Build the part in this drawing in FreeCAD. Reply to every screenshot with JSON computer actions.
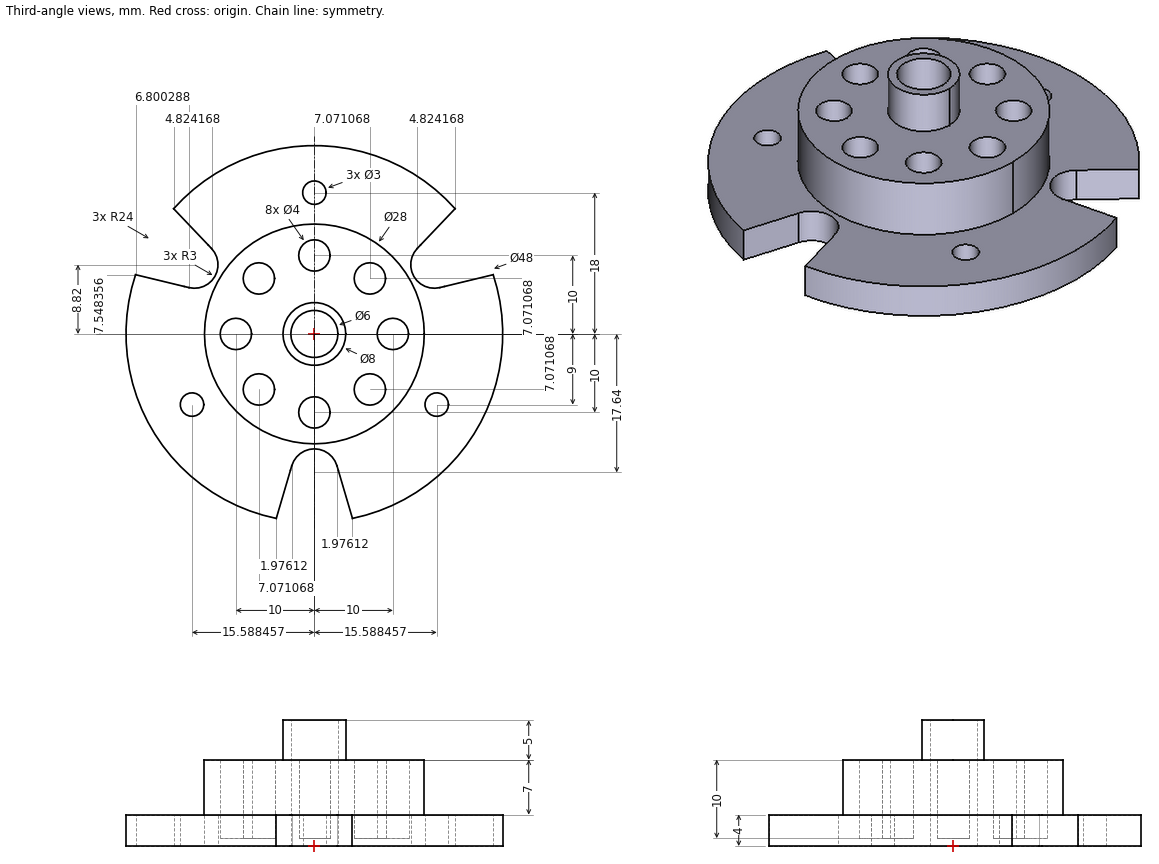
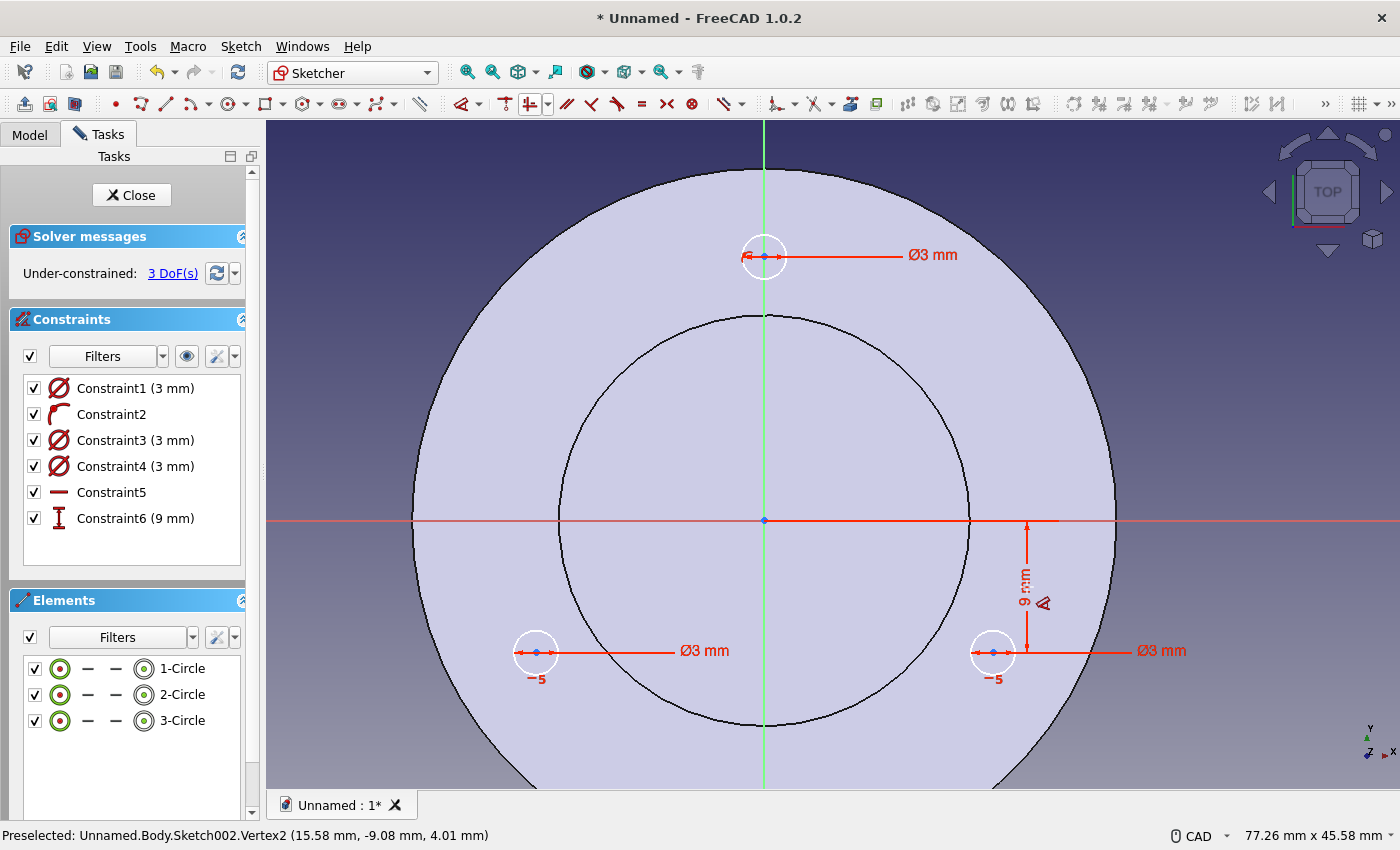
{"action": "left_click", "coordinate": [764, 257]}
{"action": "left_click", "coordinate": [798, 389]}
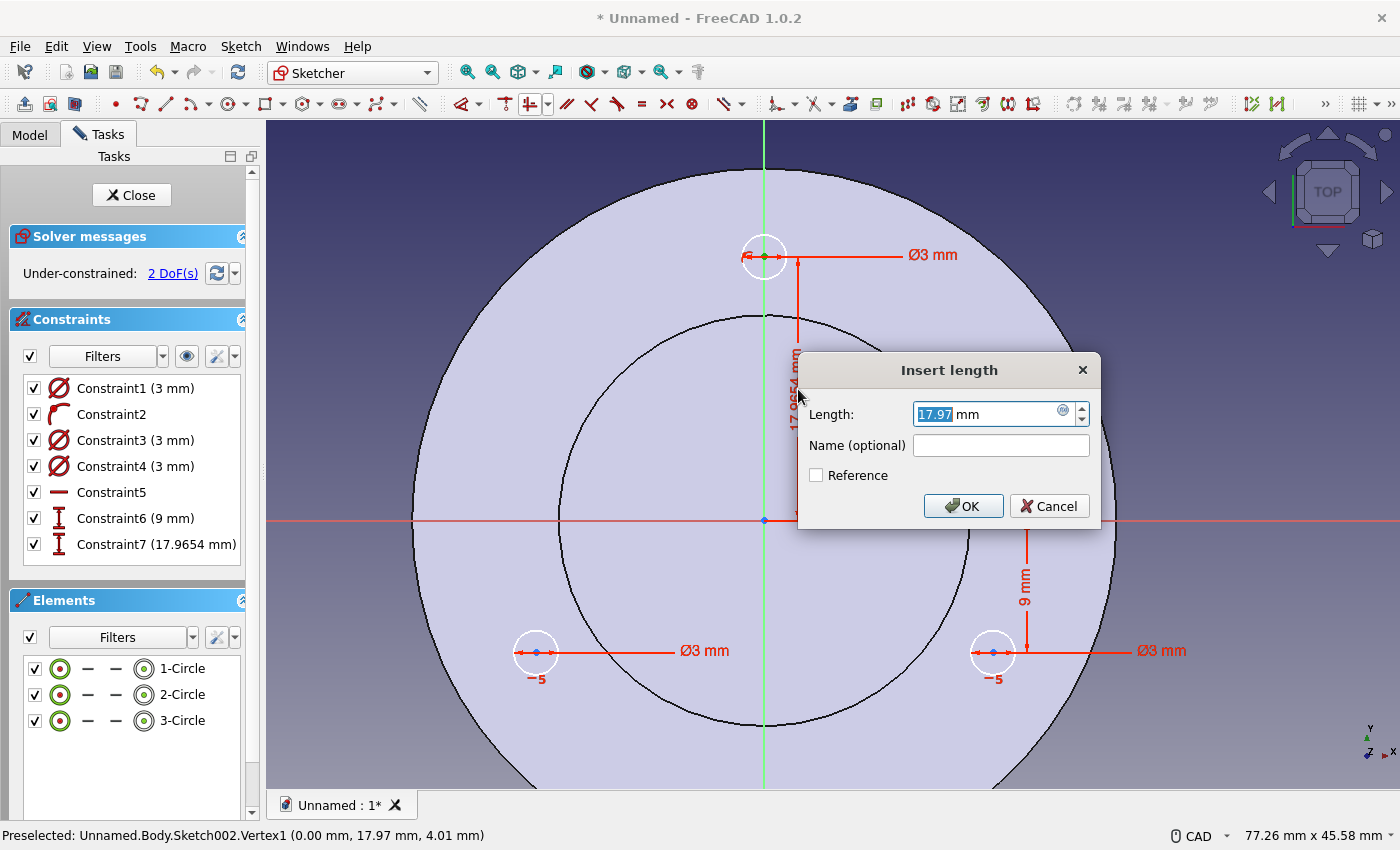
{"action": "type", "text": "18"}
{"action": "key", "text": "Return"}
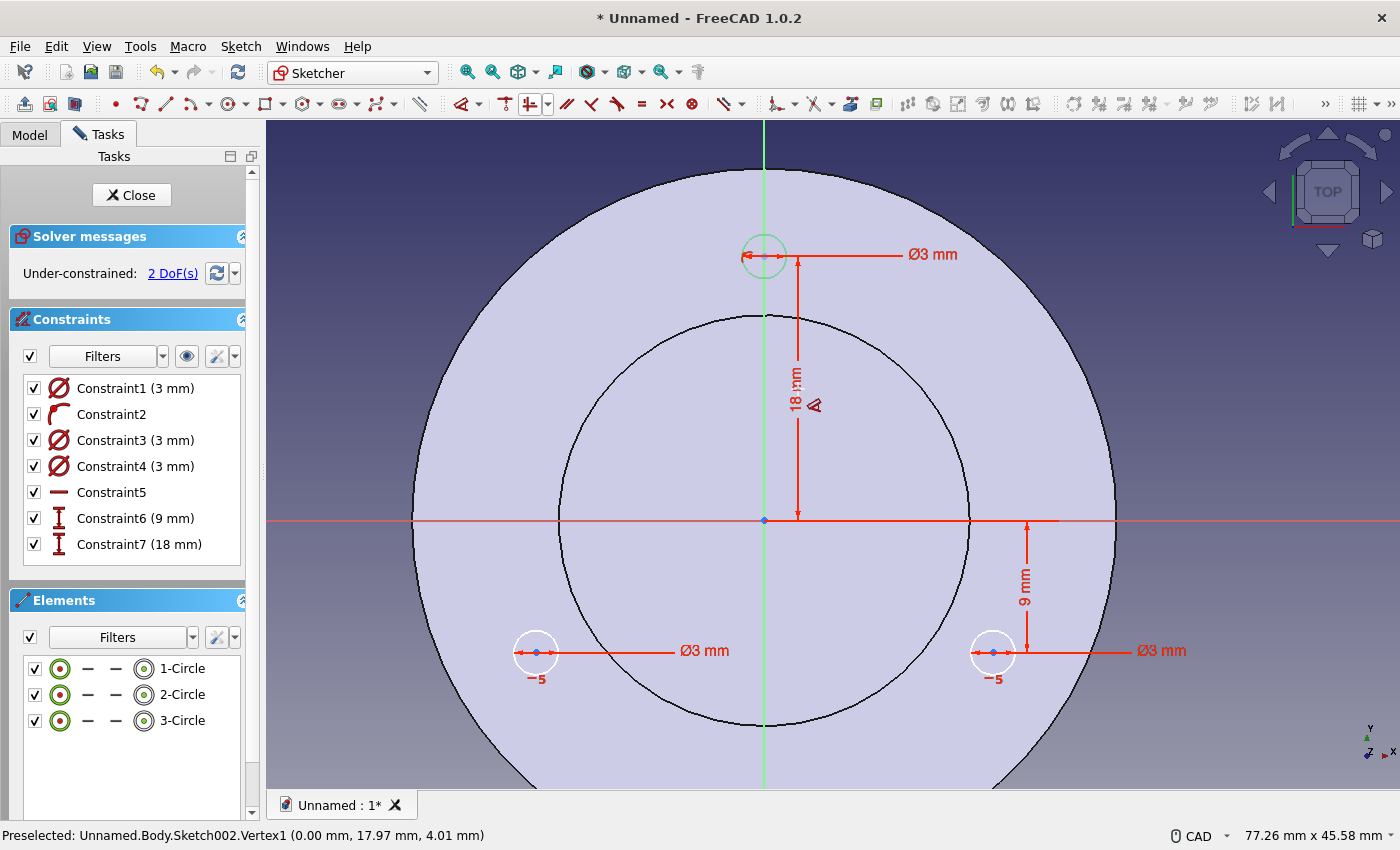
{"action": "left_click", "coordinate": [993, 653]}
{"action": "left_click", "coordinate": [879, 687]}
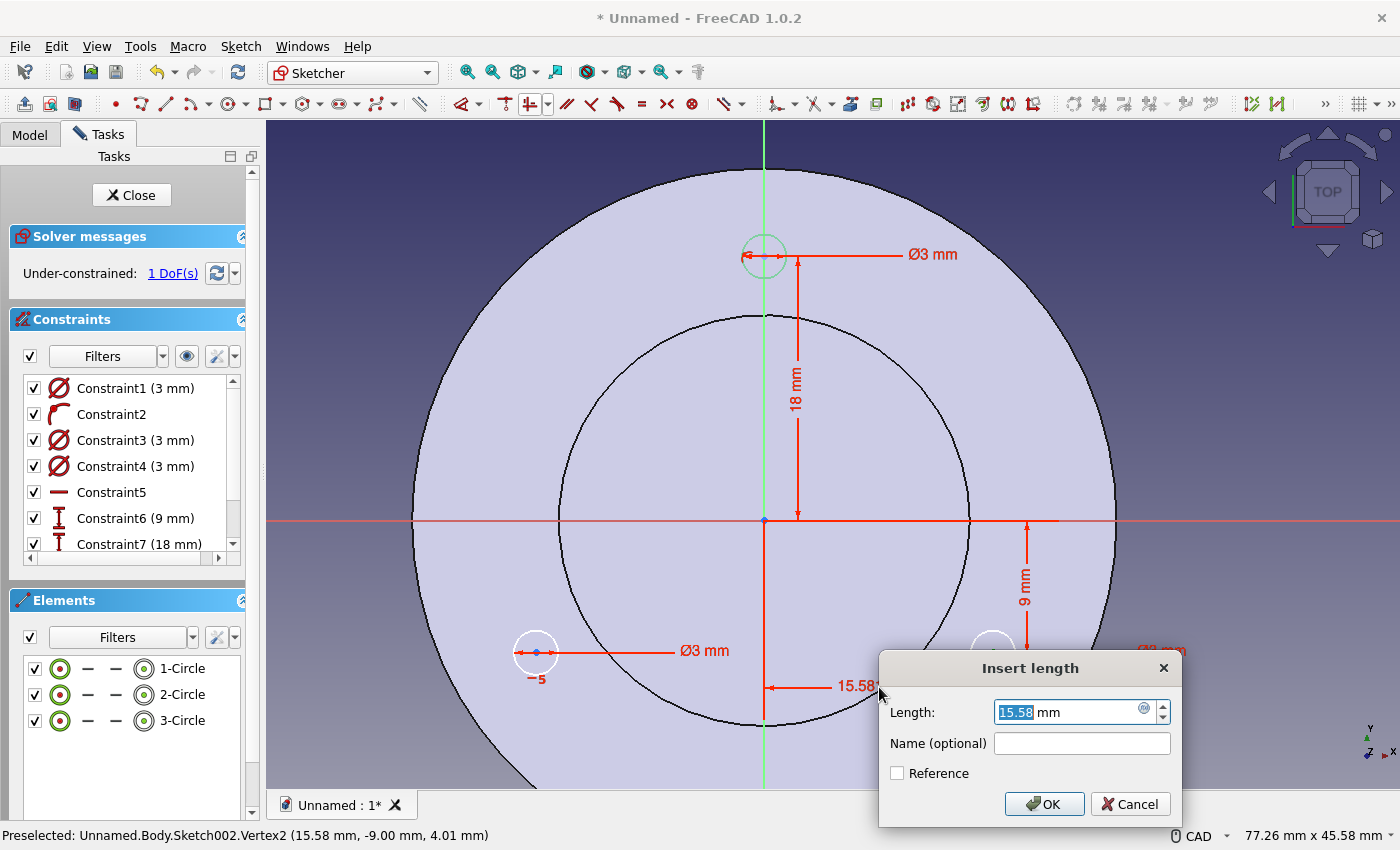
{"action": "type", "text": "15.588457"}
{"action": "key", "text": "Return"}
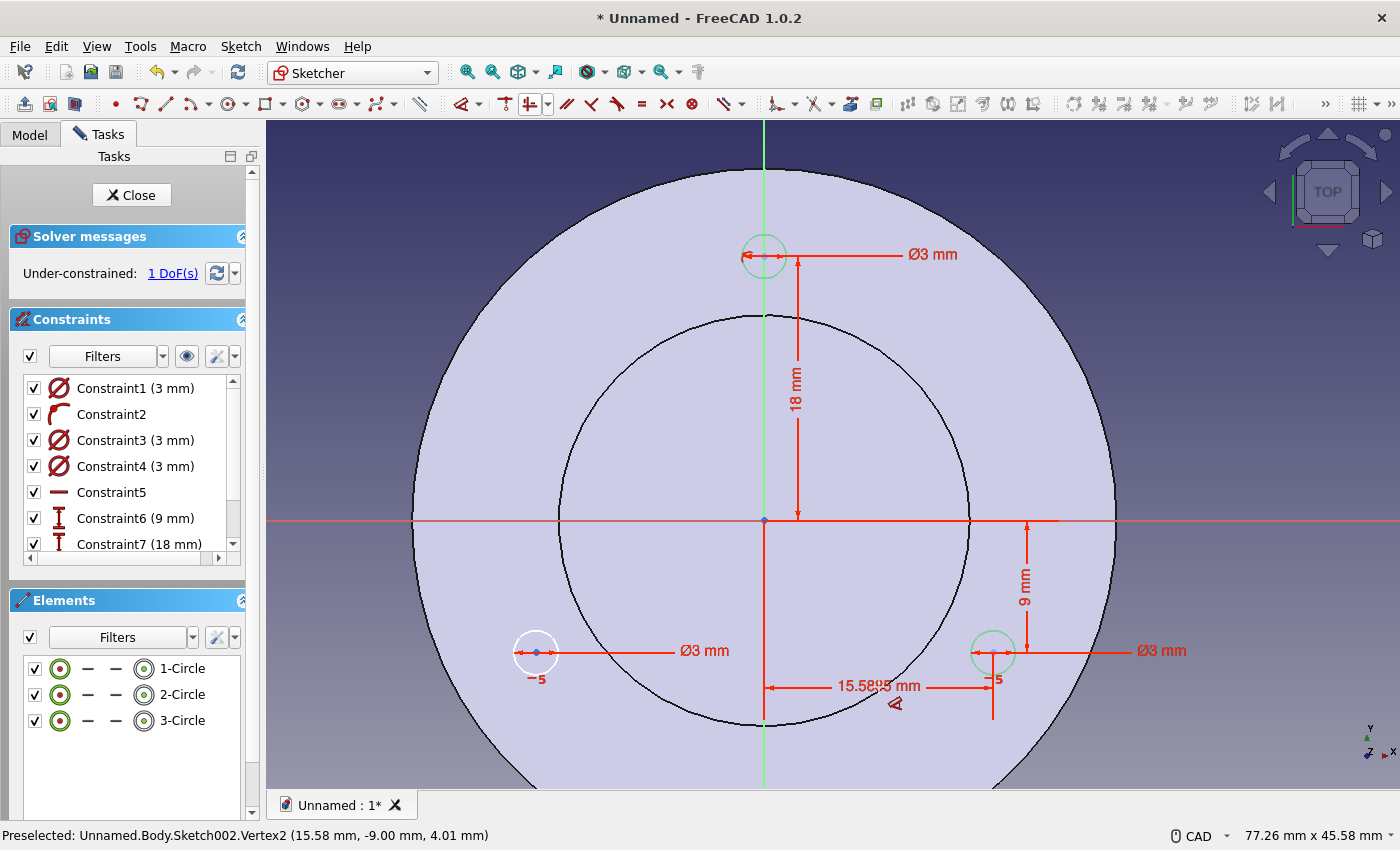
{"action": "left_click", "coordinate": [536, 653]}
{"action": "left_click", "coordinate": [650, 687]}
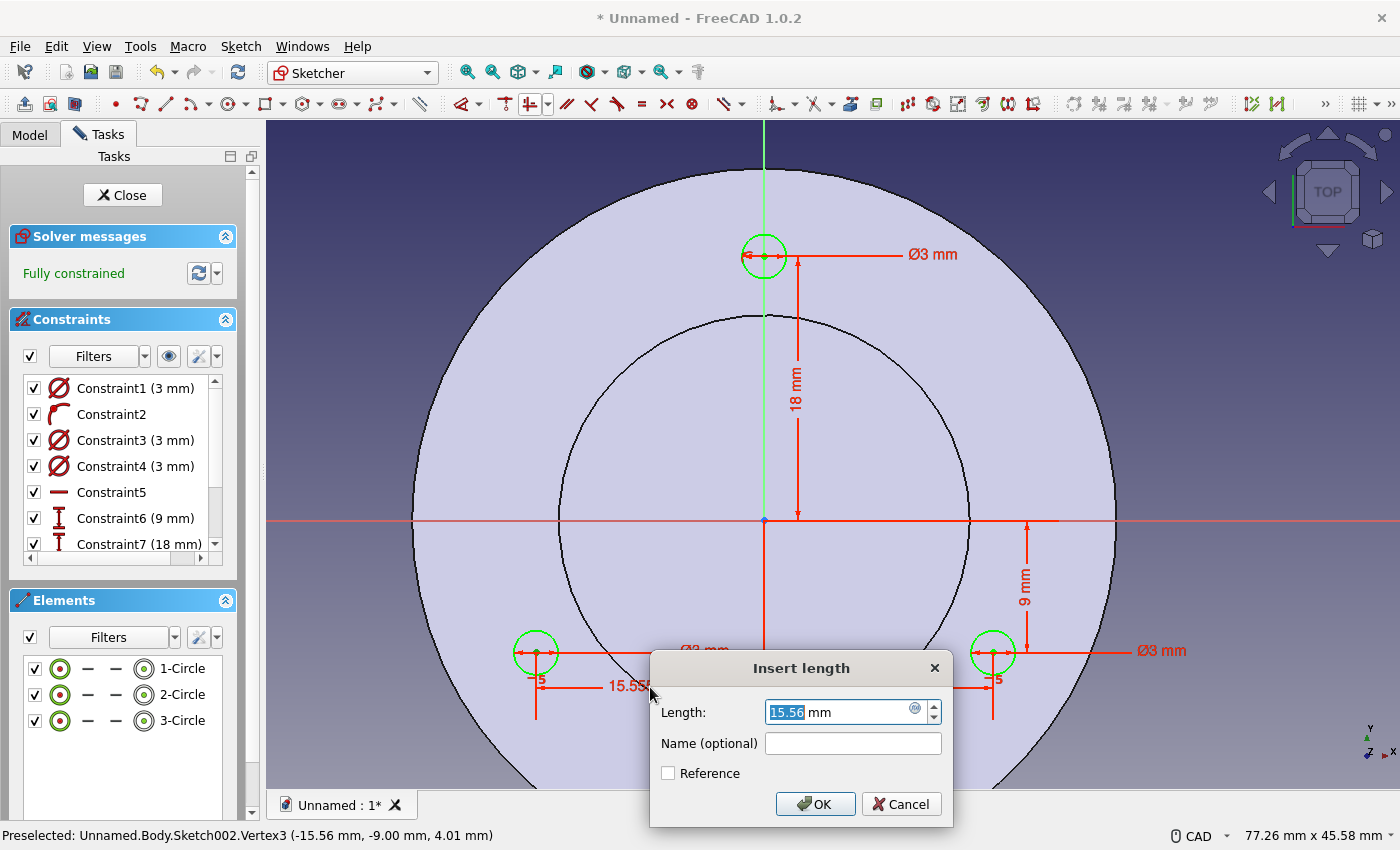
{"action": "type", "text": "15.588457"}
{"action": "key", "text": "Return"}
{"action": "key", "text": "Escape"}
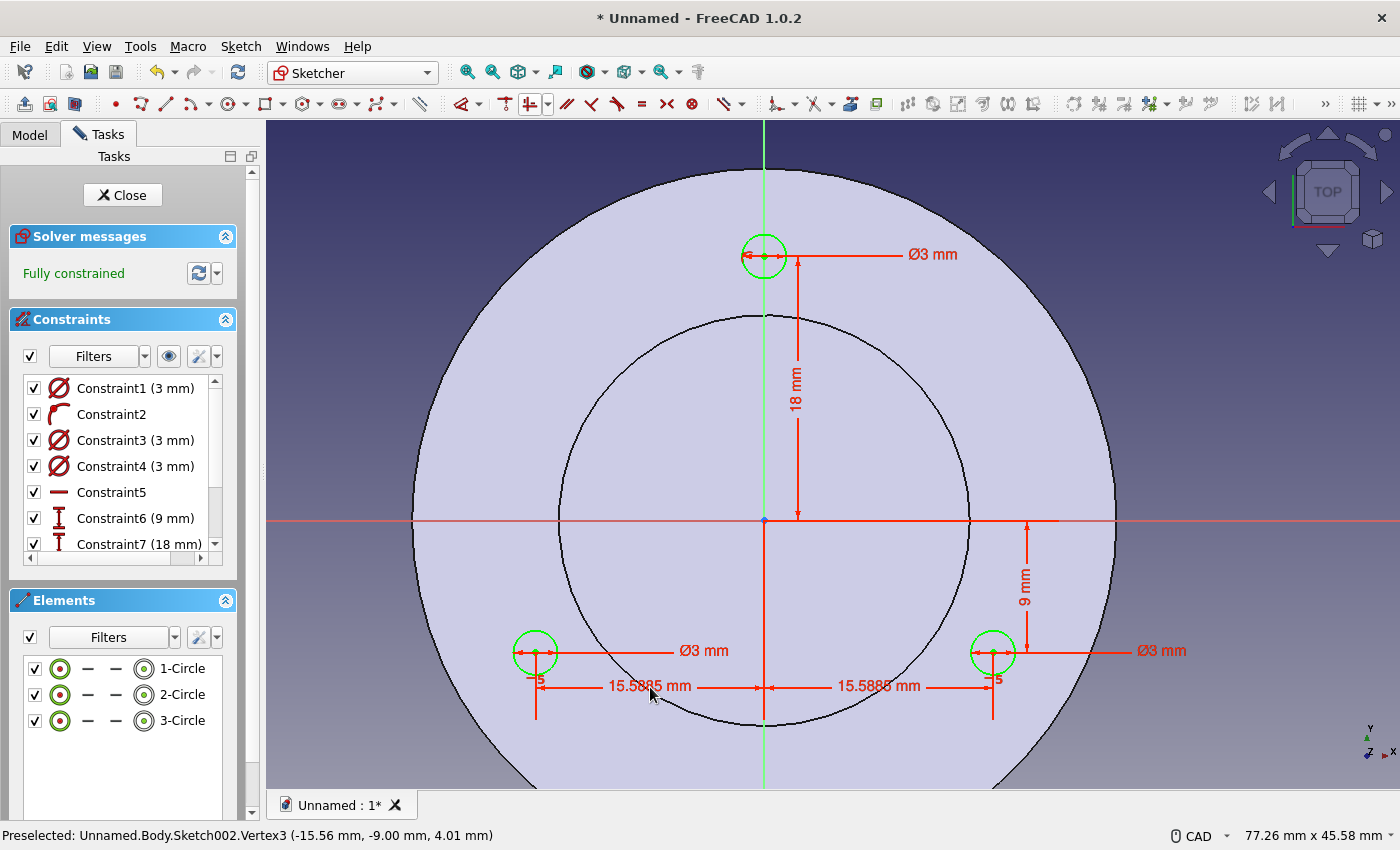
{"action": "left_click", "coordinate": [123, 195]}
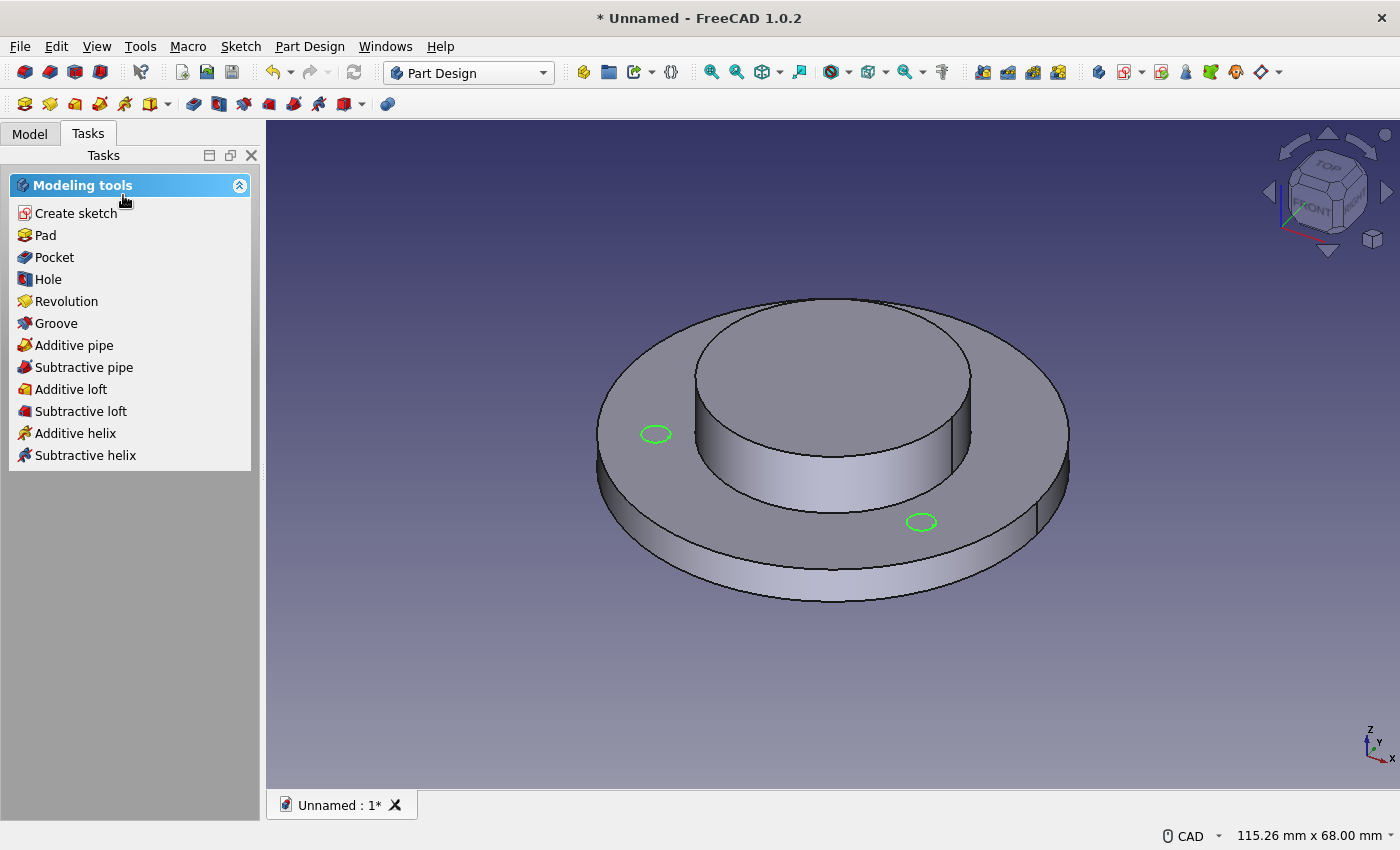
{"action": "left_click", "coordinate": [194, 104]}